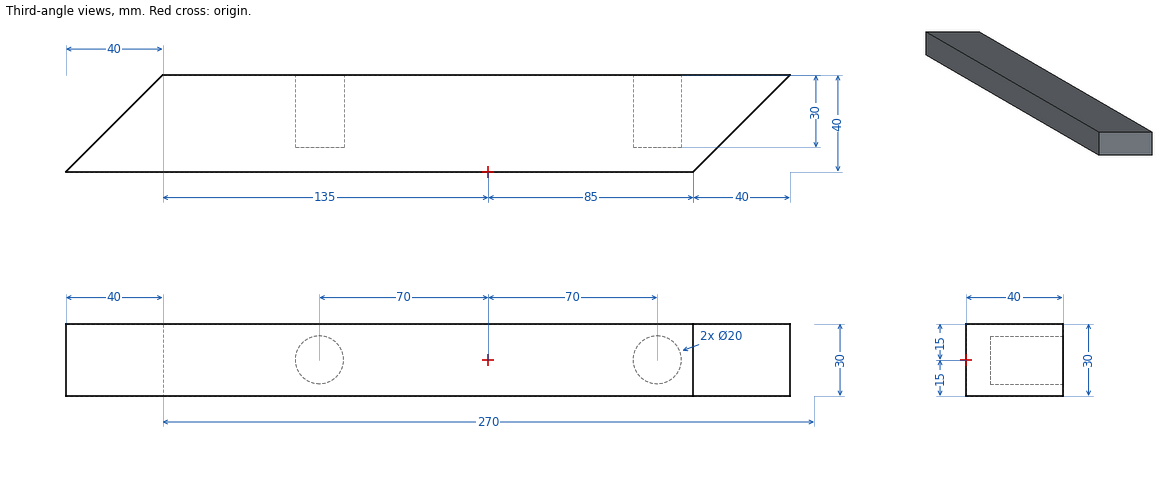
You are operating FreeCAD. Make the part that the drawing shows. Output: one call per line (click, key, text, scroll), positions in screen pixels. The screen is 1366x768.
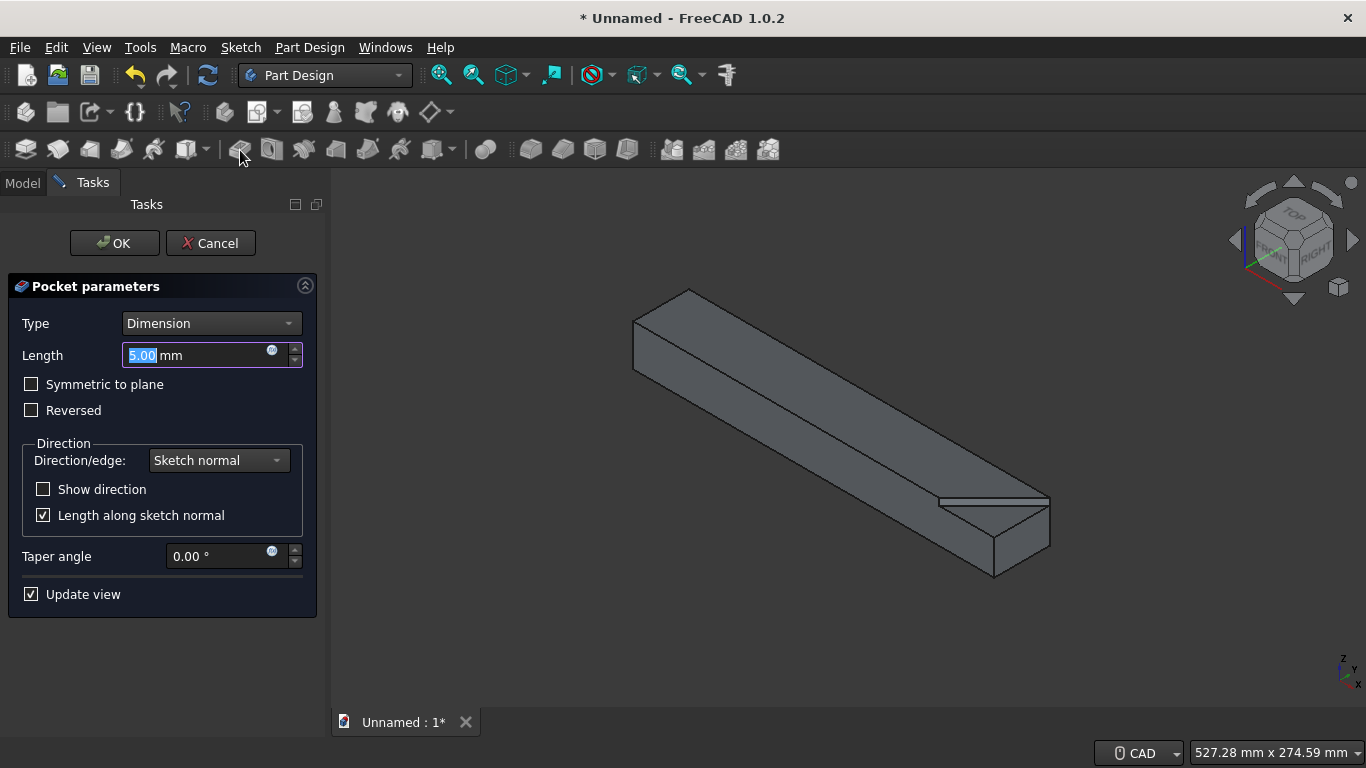
click(212, 324)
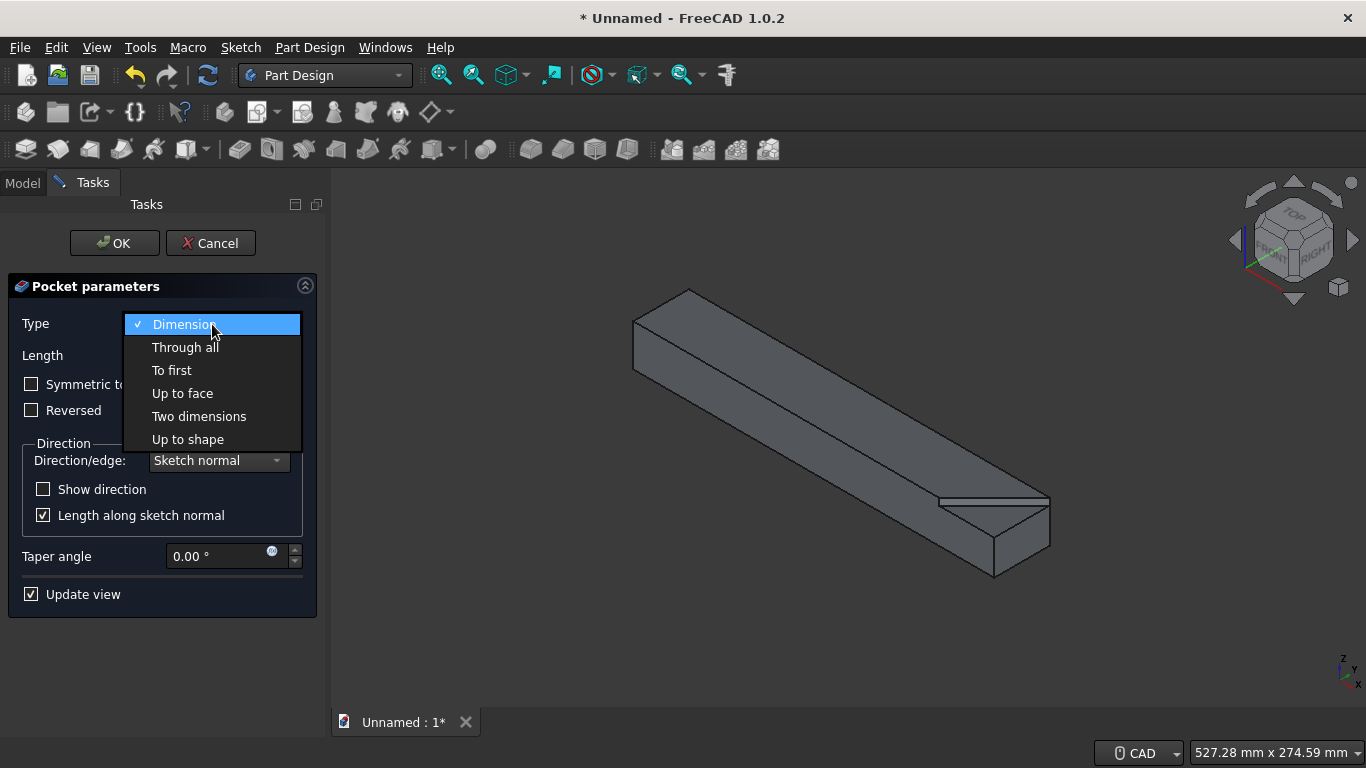
click(212, 348)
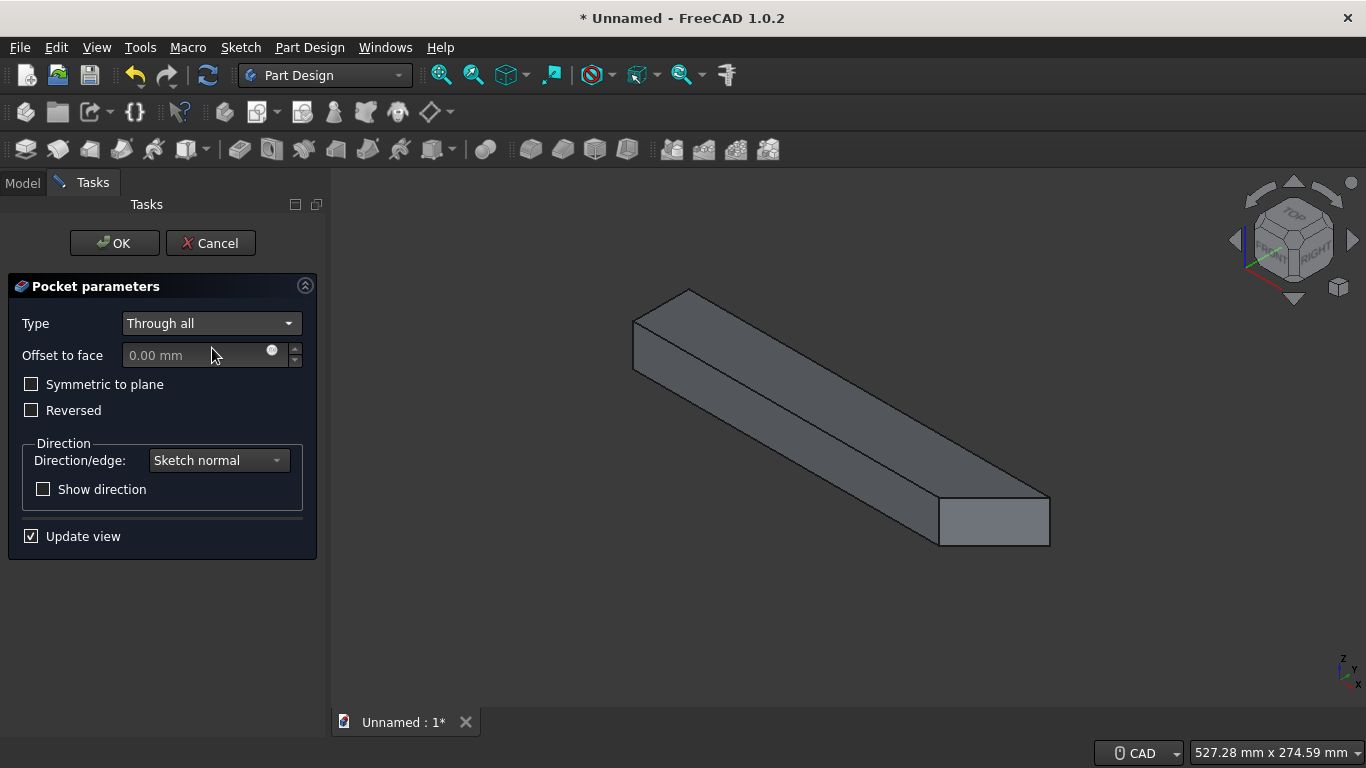
click(115, 243)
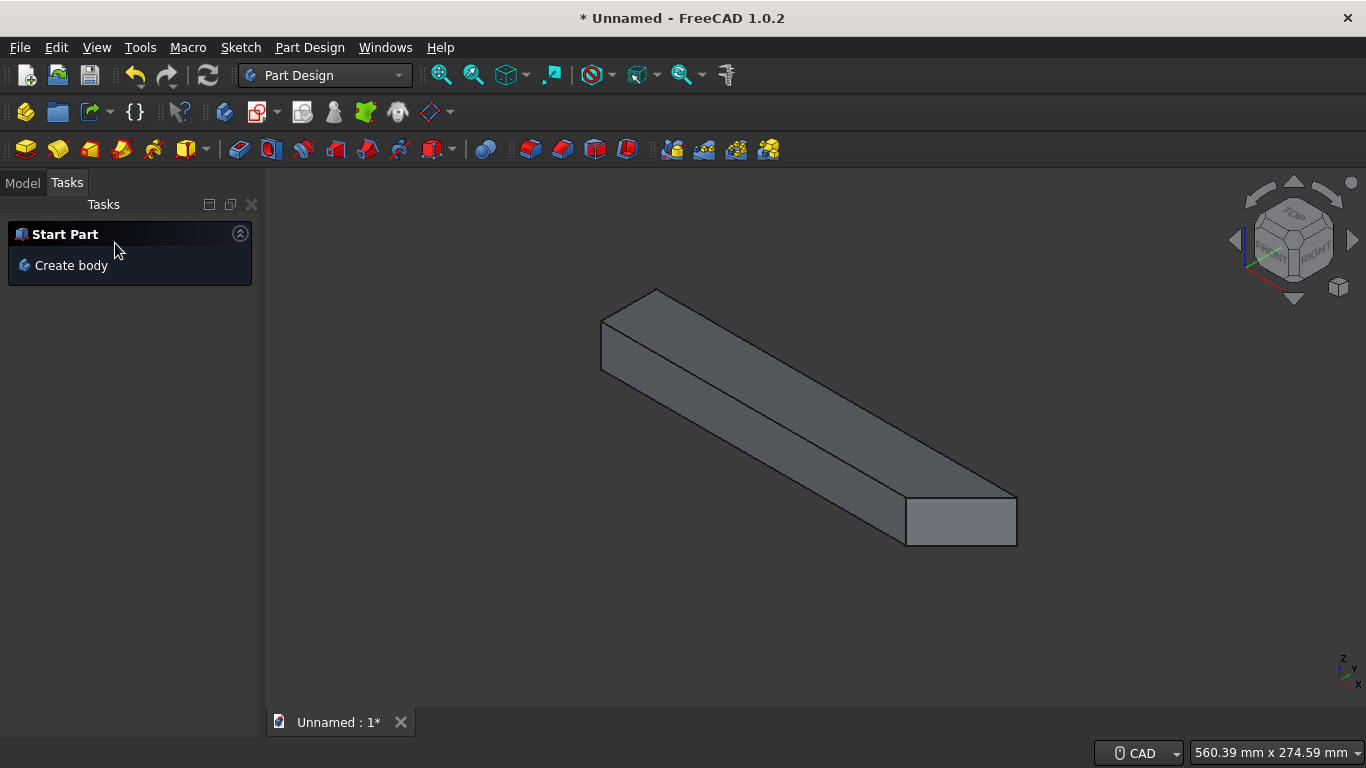
key(6)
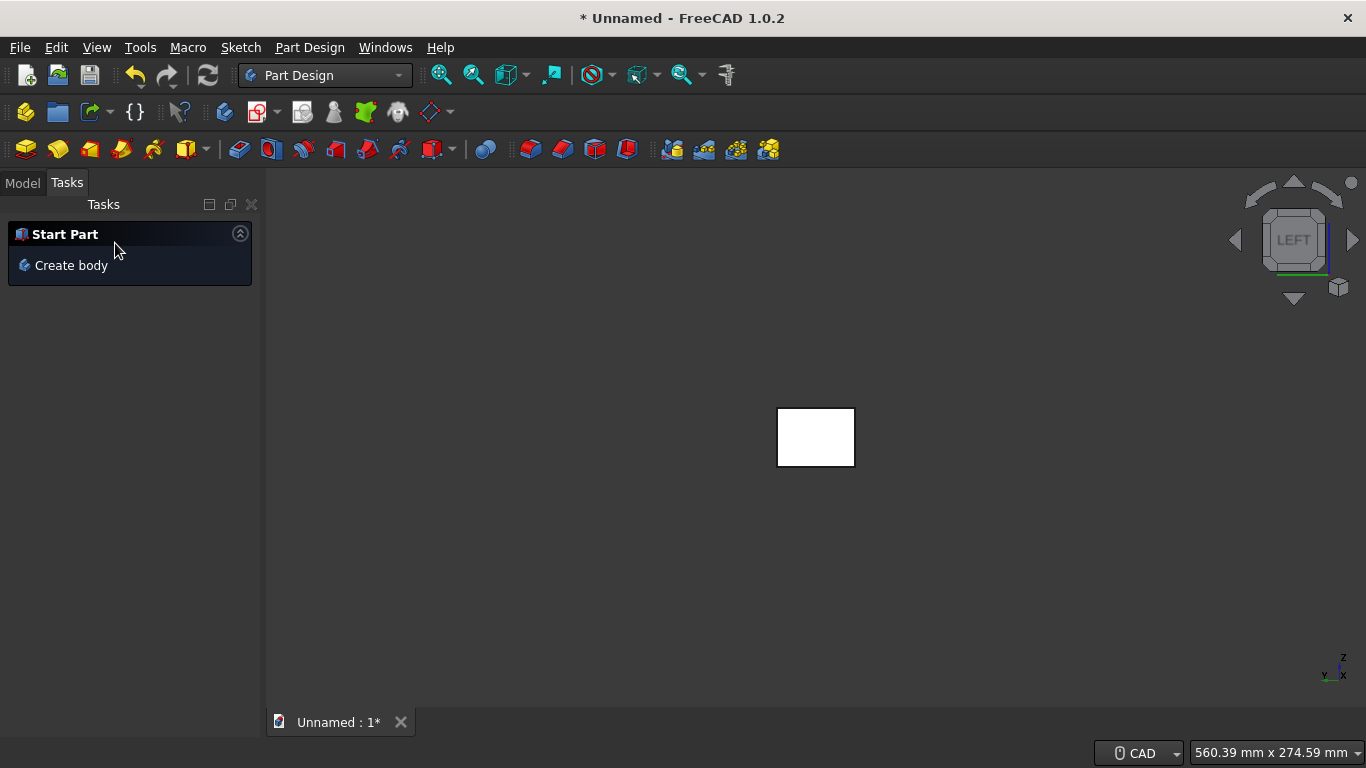
click(442, 76)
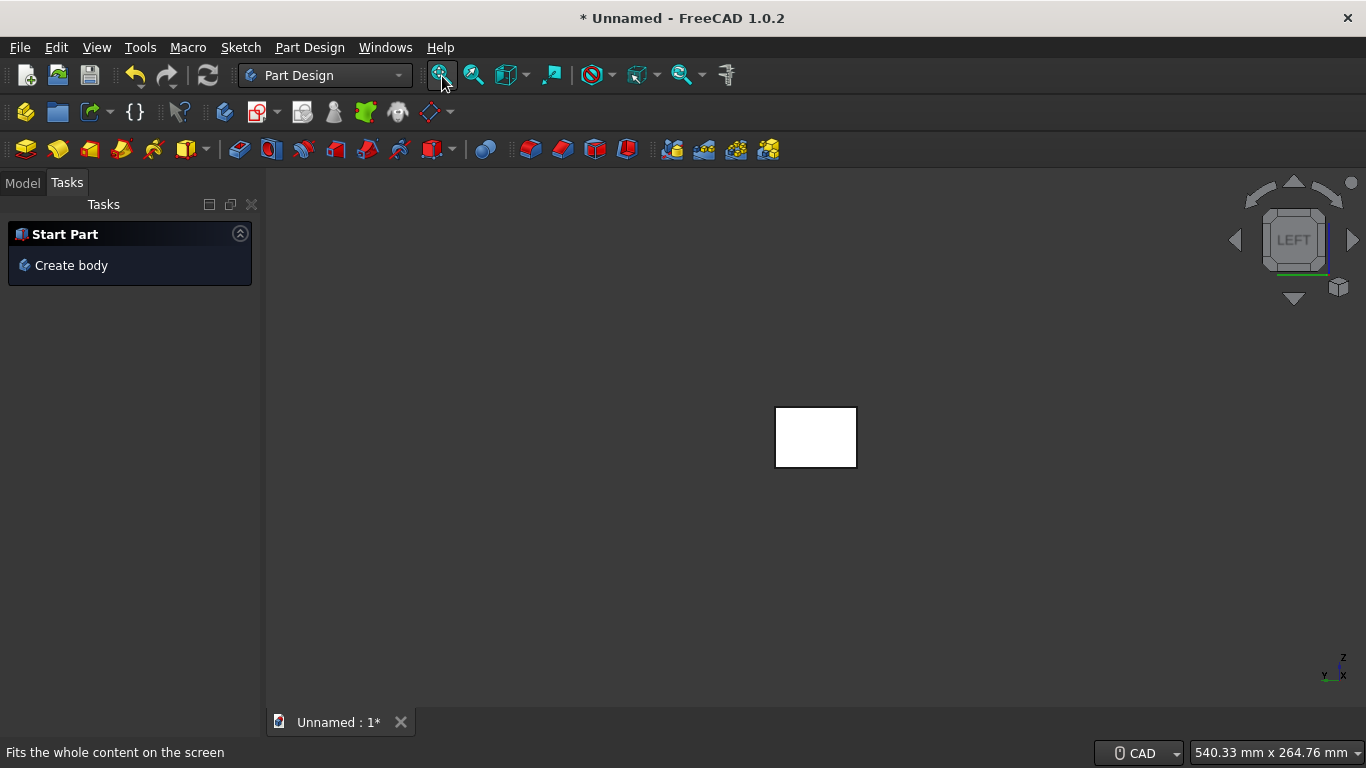
click(816, 436)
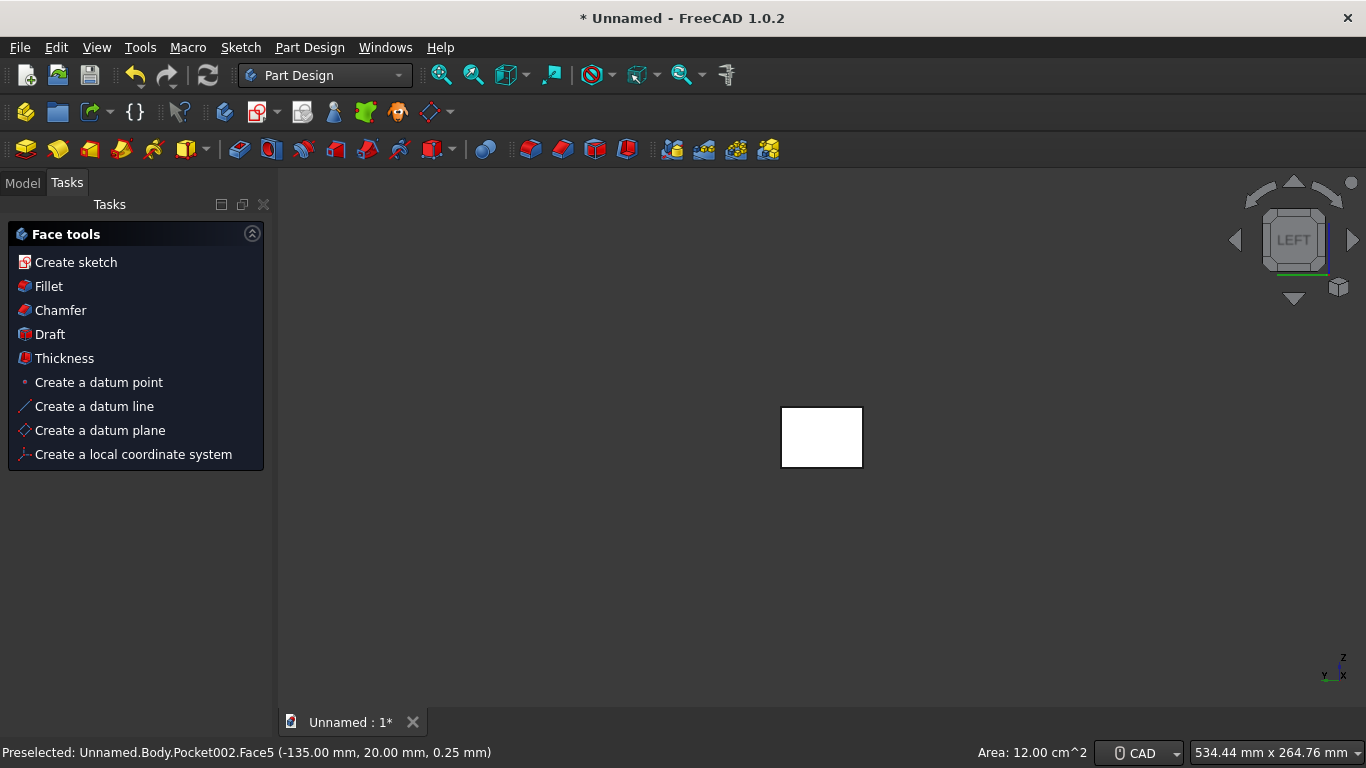
click(258, 112)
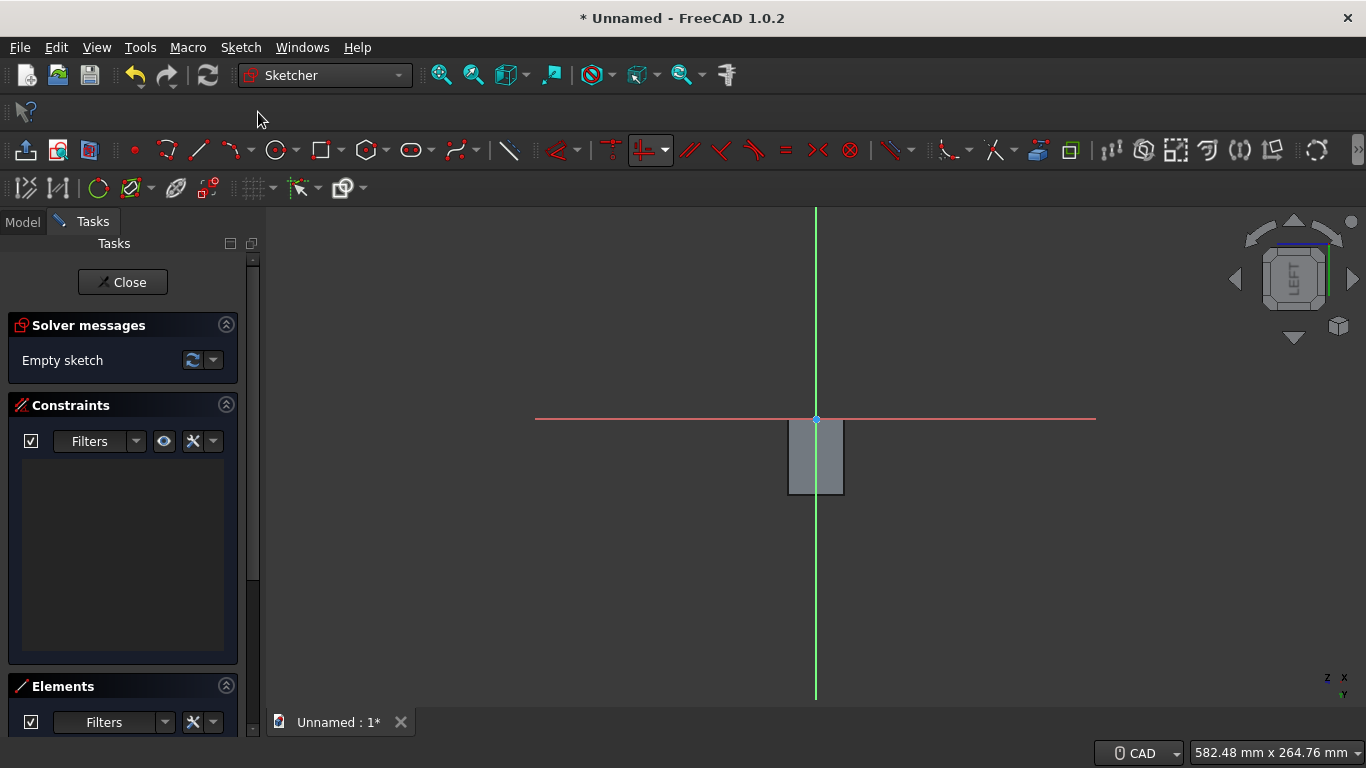
scroll(838, 457, up, 7)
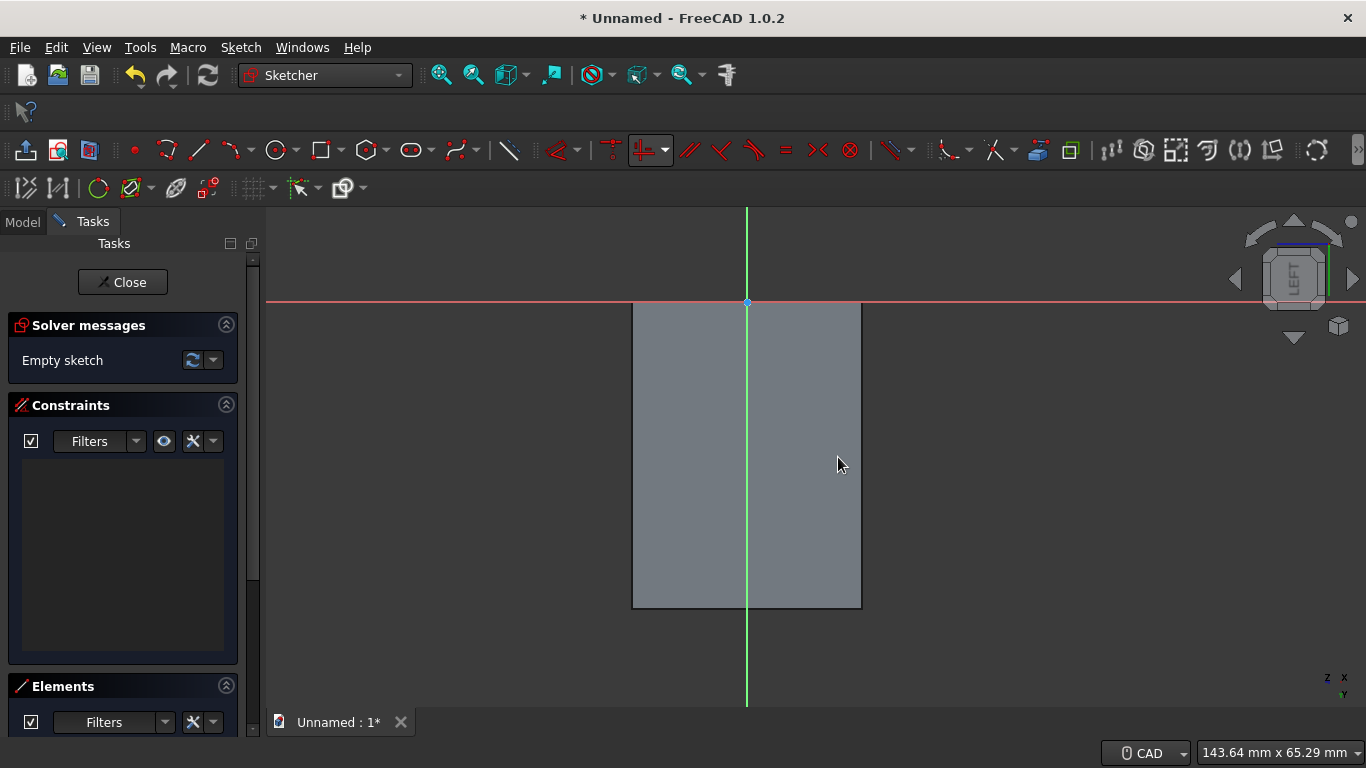
click(322, 150)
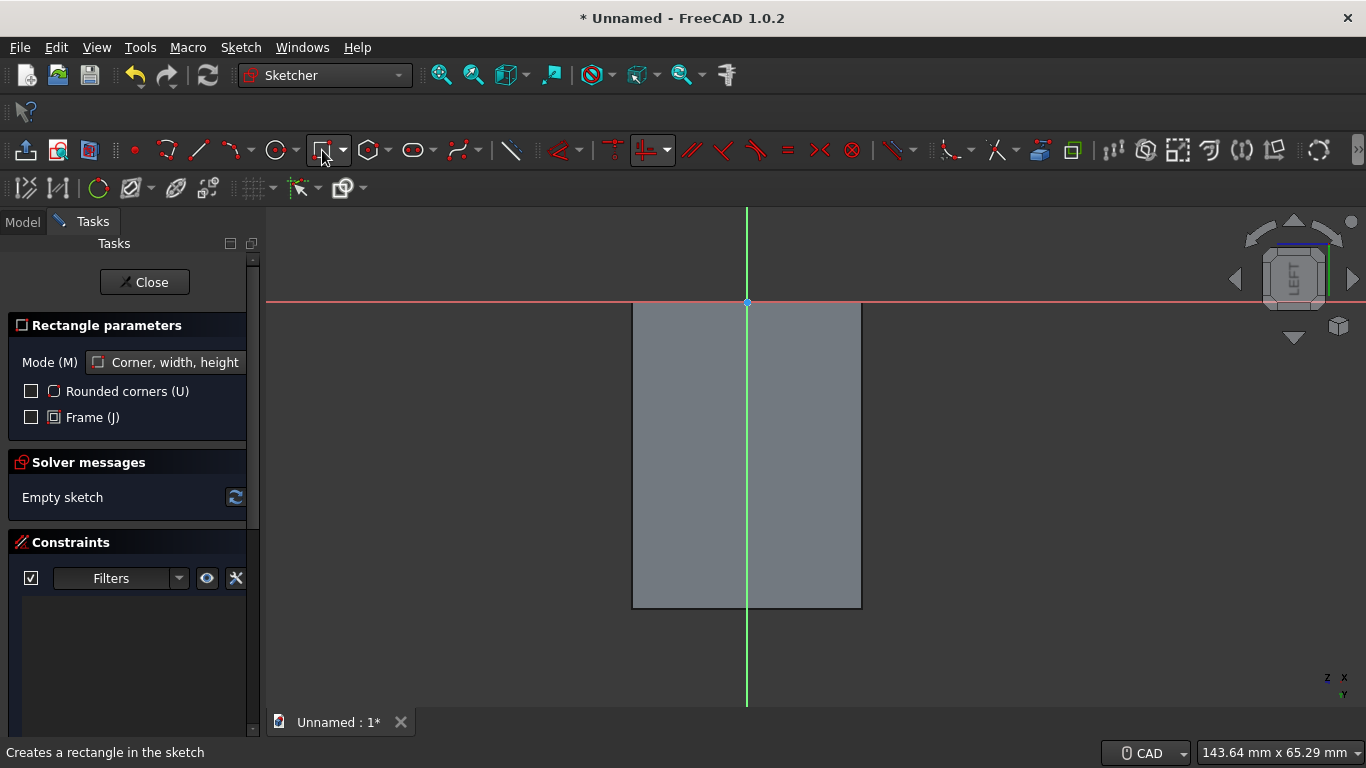
click(632, 302)
click(862, 609)
key(Escape)